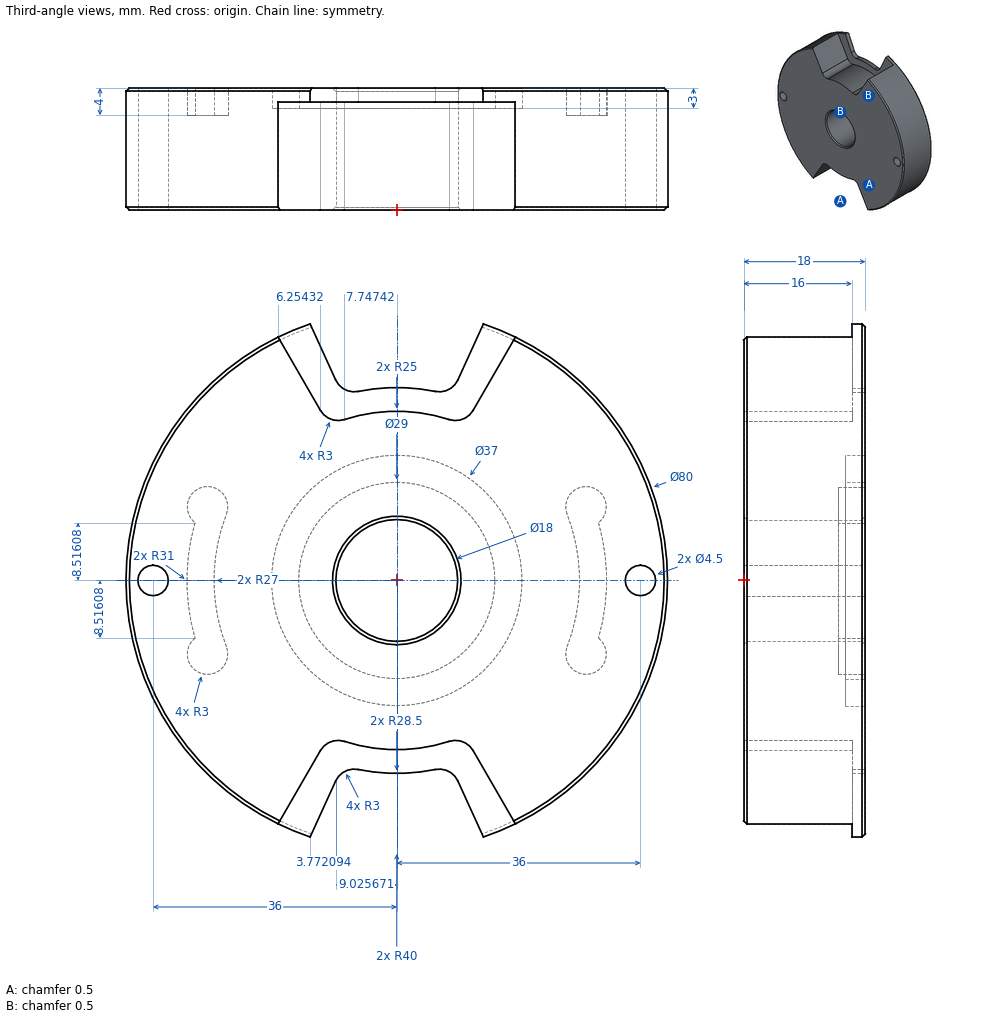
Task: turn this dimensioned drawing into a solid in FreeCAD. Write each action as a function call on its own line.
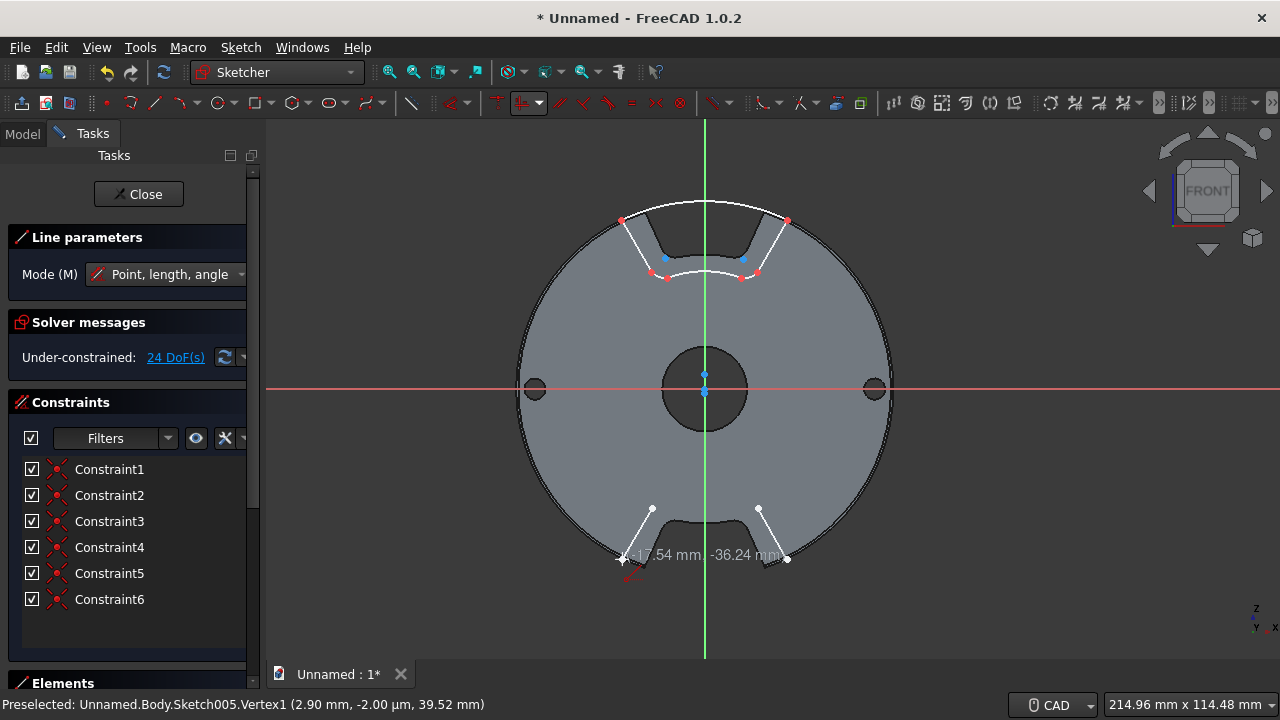
click(180, 104)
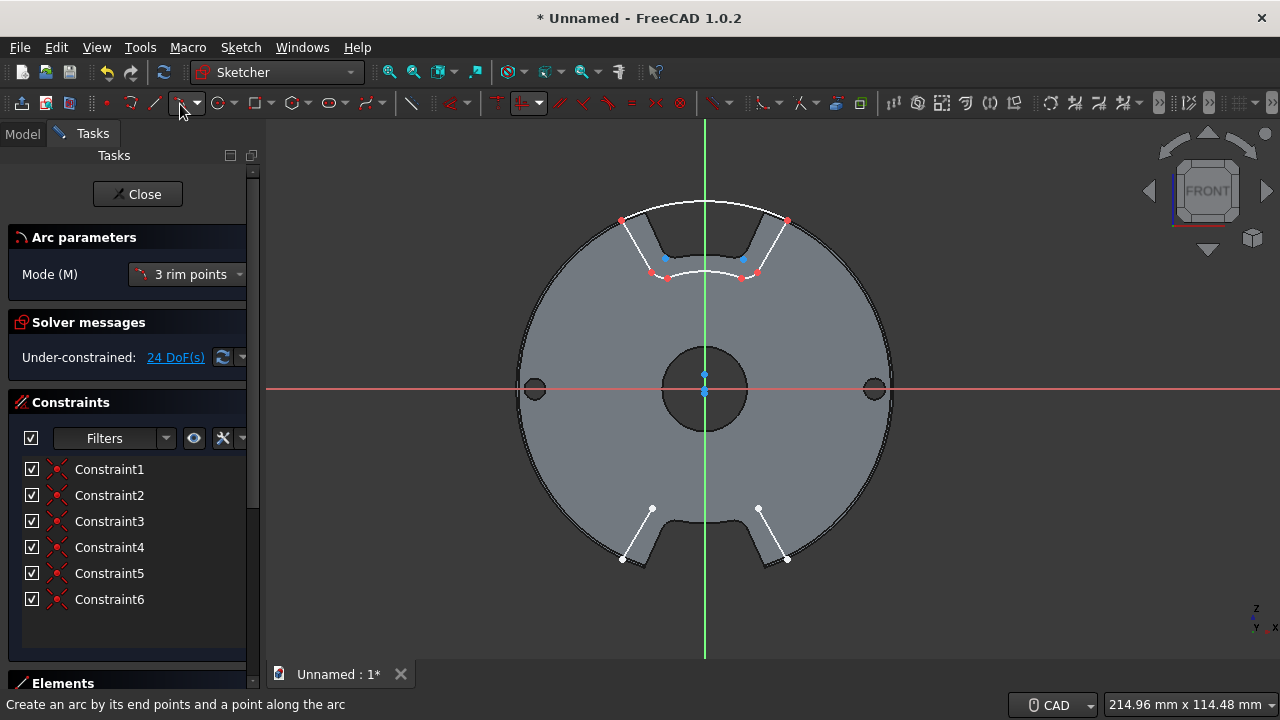
click(758, 509)
click(741, 501)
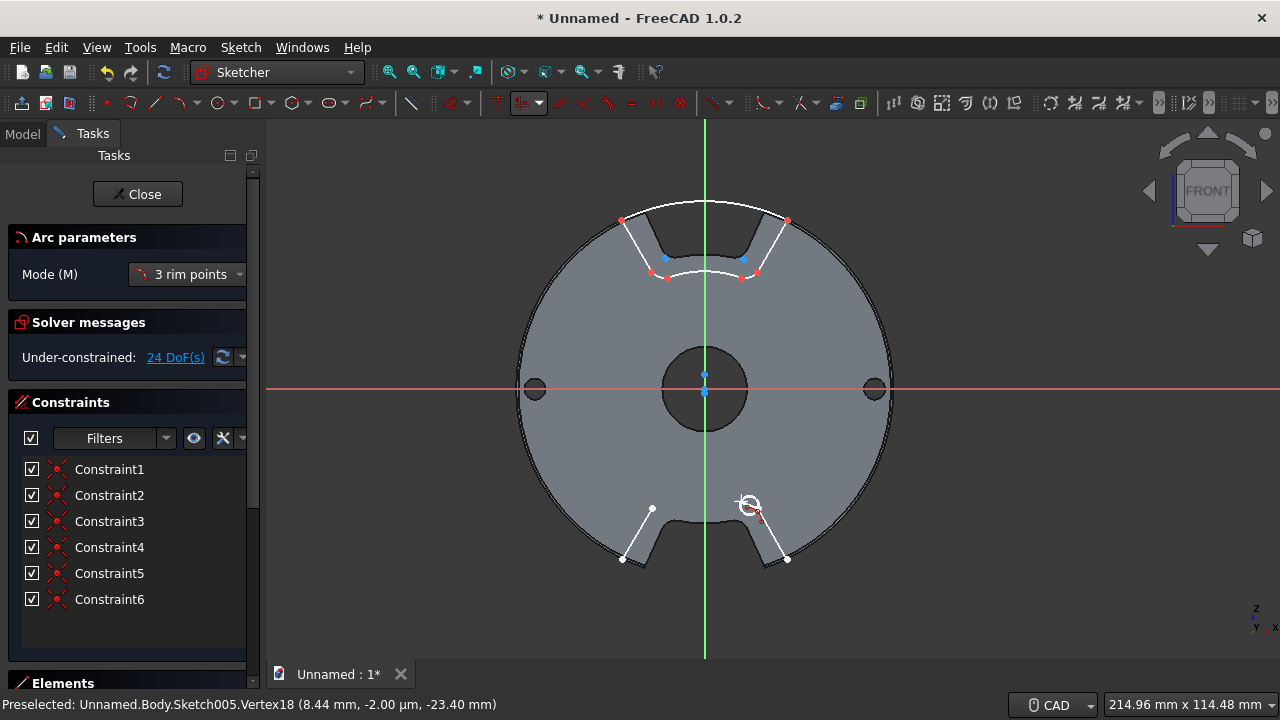
scroll(751, 501, up, 9)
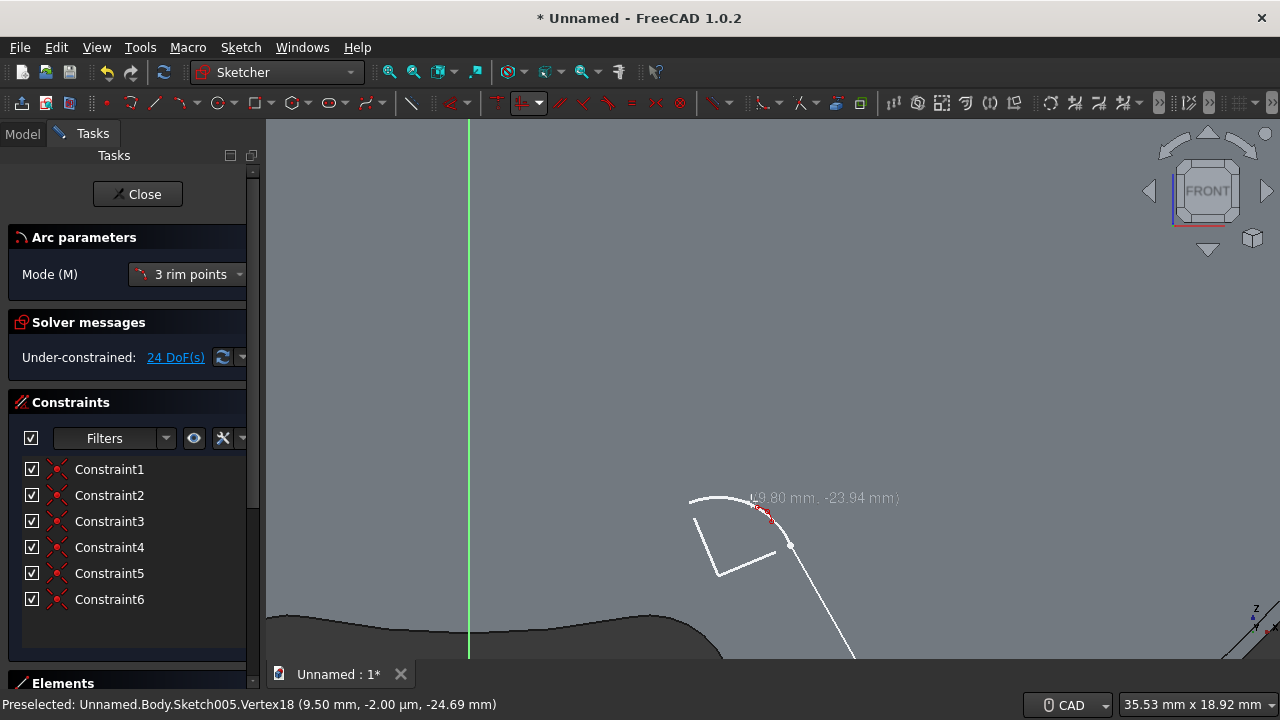
click(747, 500)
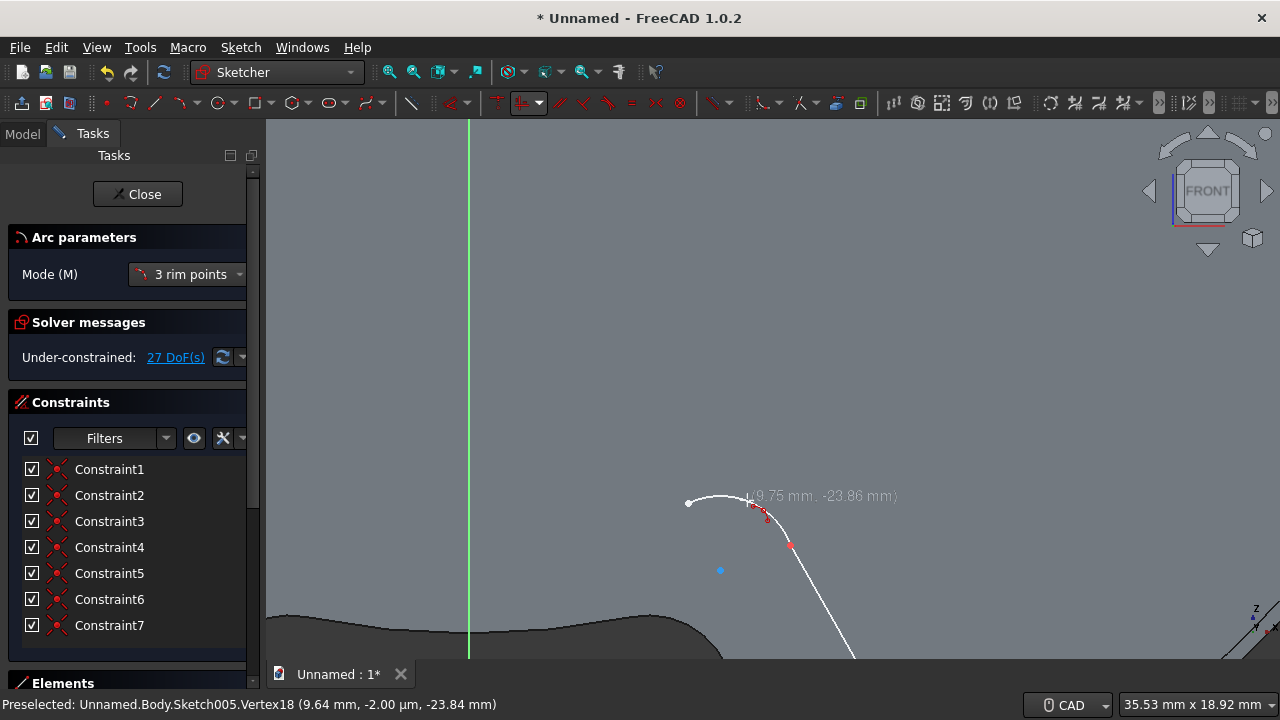
scroll(751, 502, down, 9)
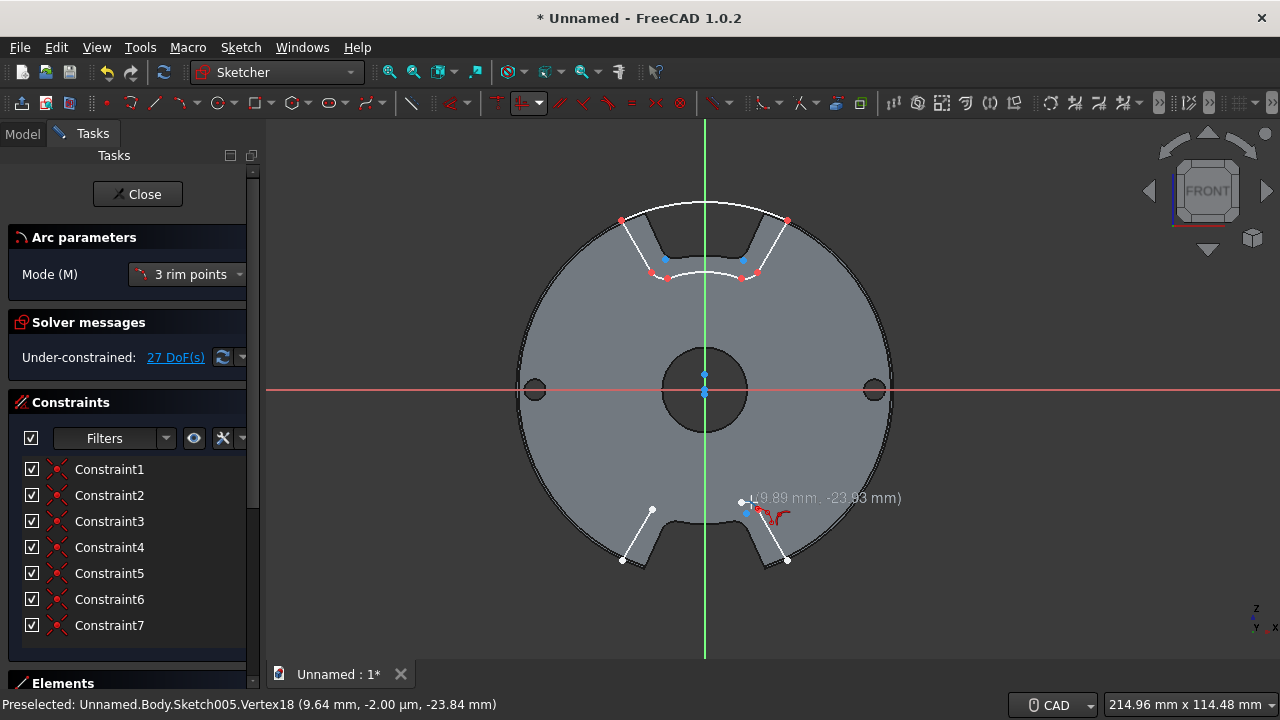
click(741, 503)
click(668, 502)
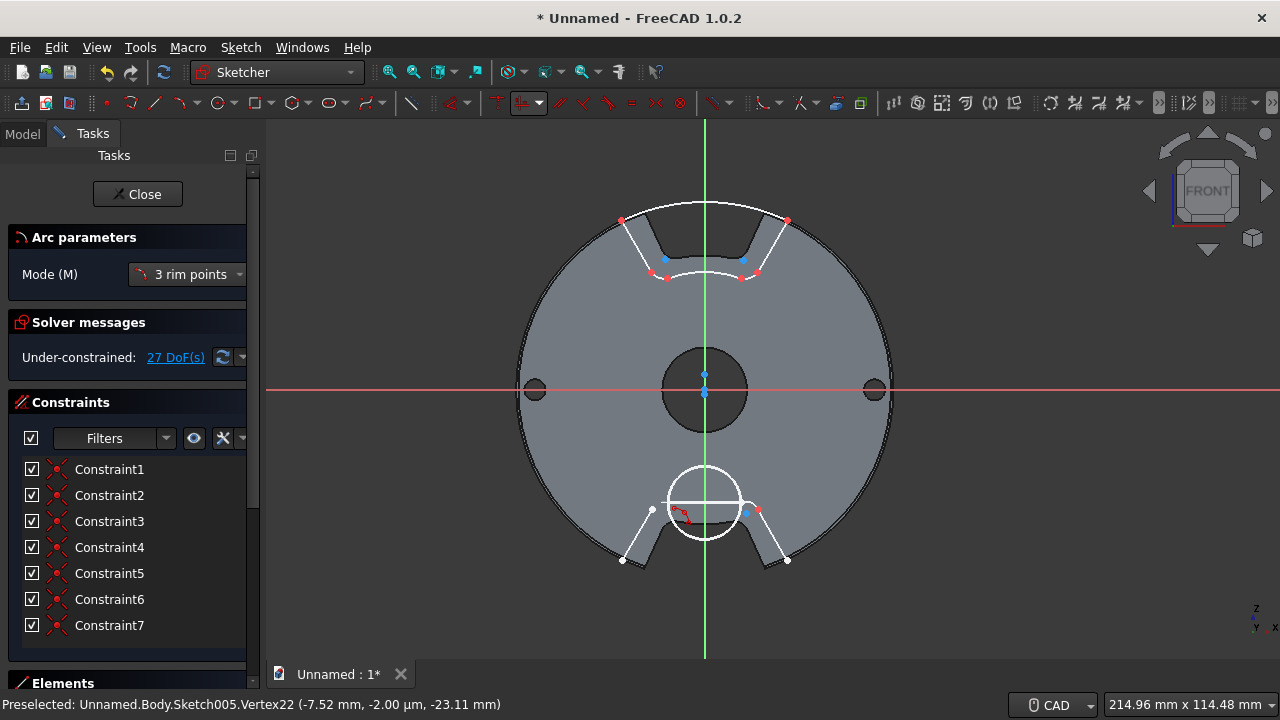
scroll(697, 508, up, 6)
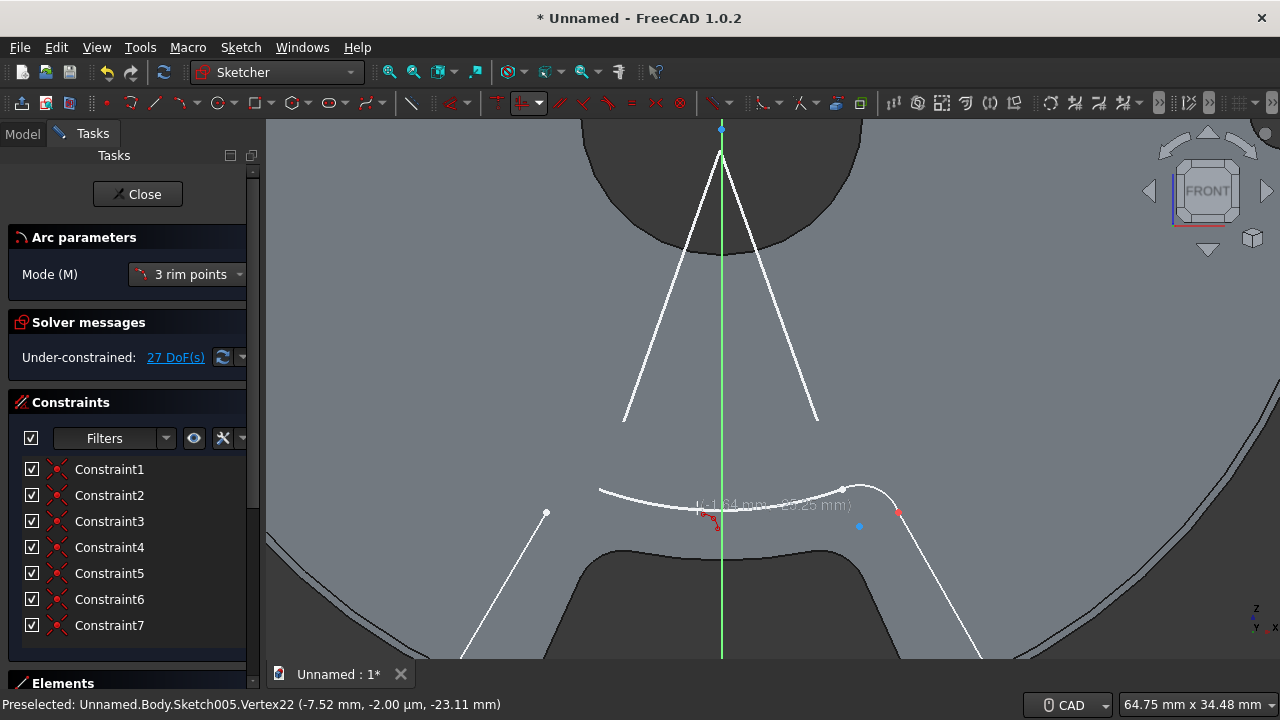
click(697, 505)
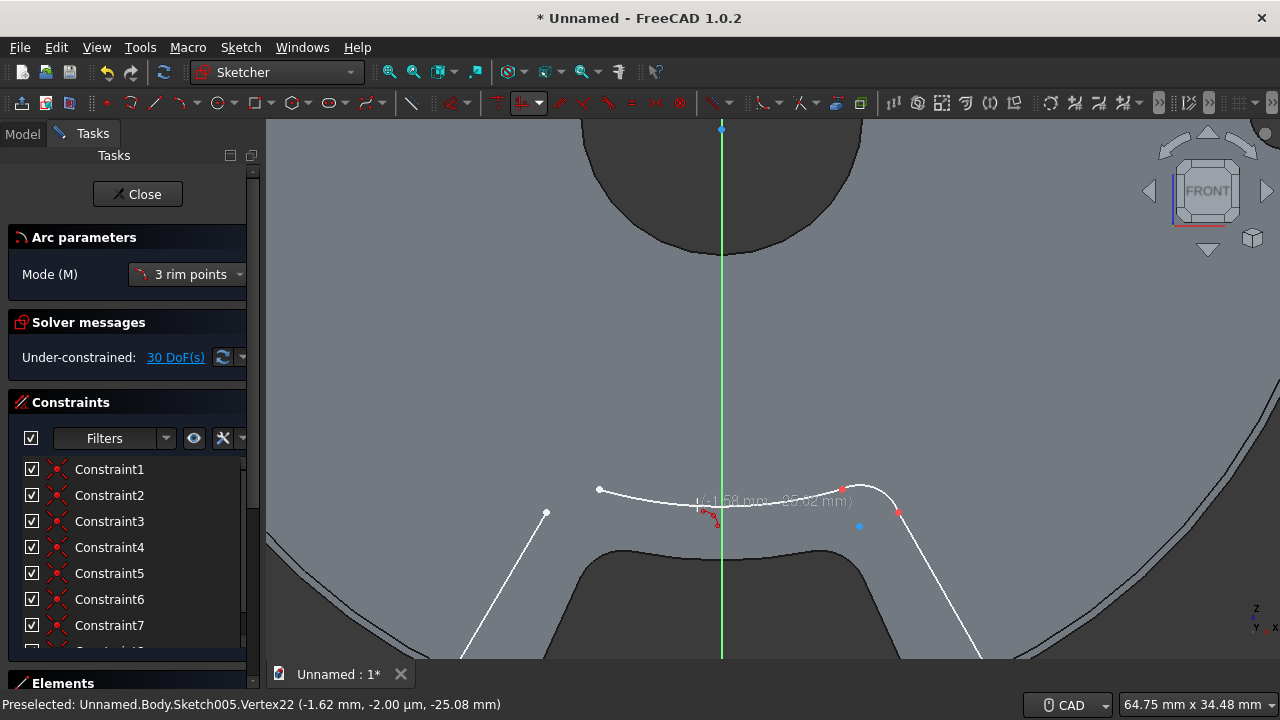
click(600, 490)
click(547, 512)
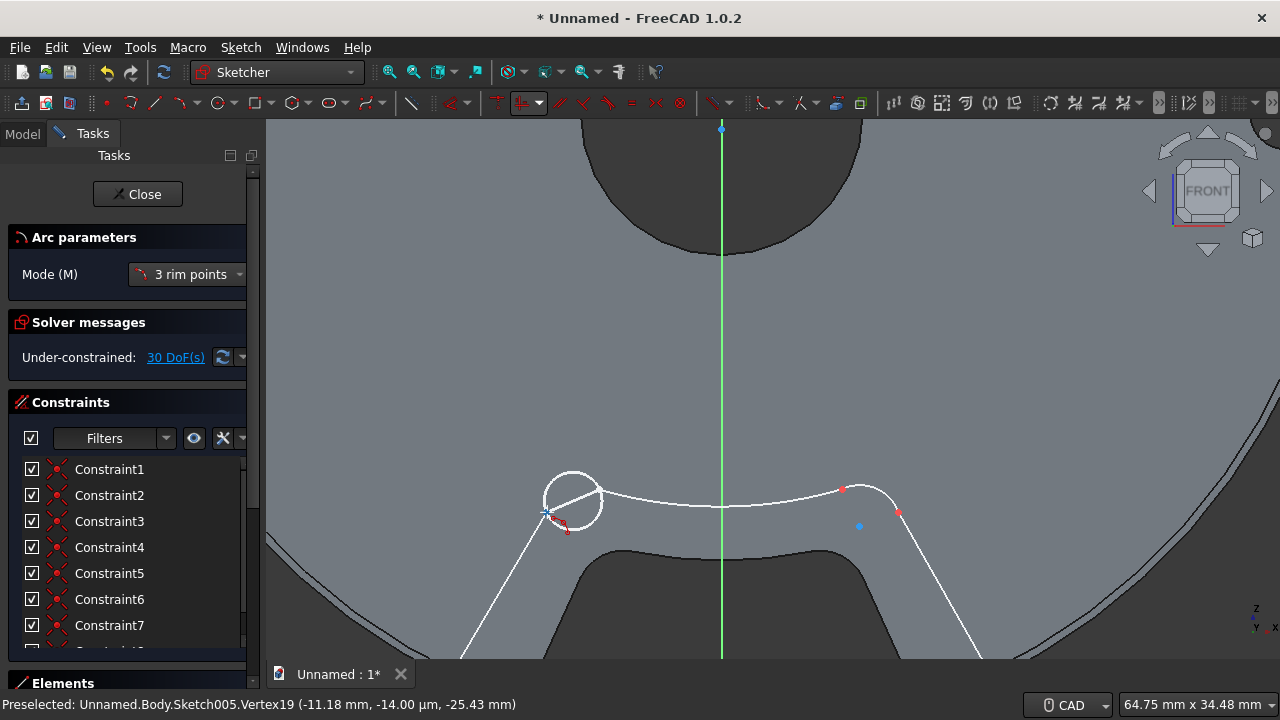
scroll(569, 487, up, 3)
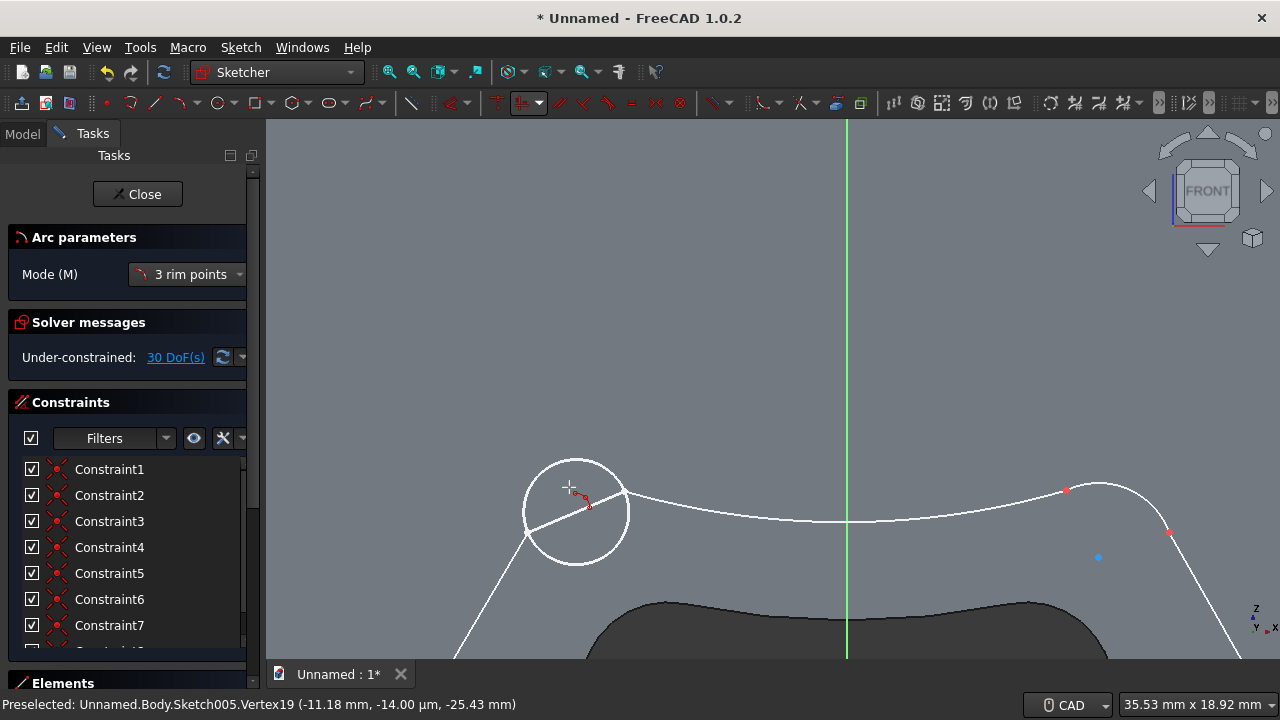
click(569, 487)